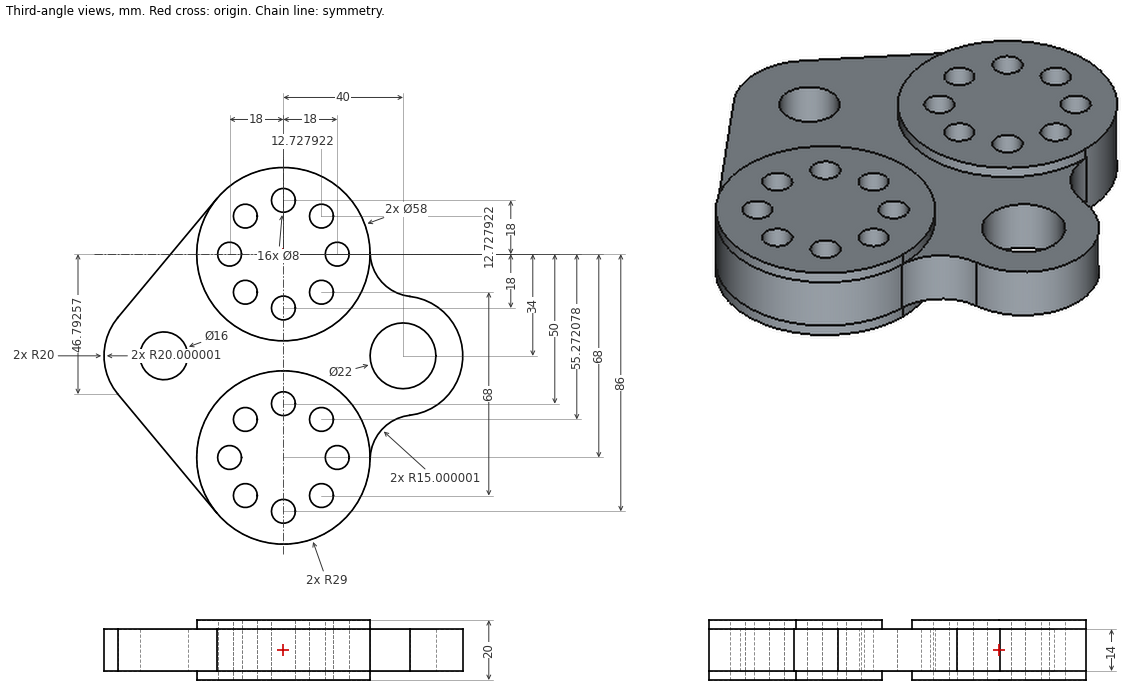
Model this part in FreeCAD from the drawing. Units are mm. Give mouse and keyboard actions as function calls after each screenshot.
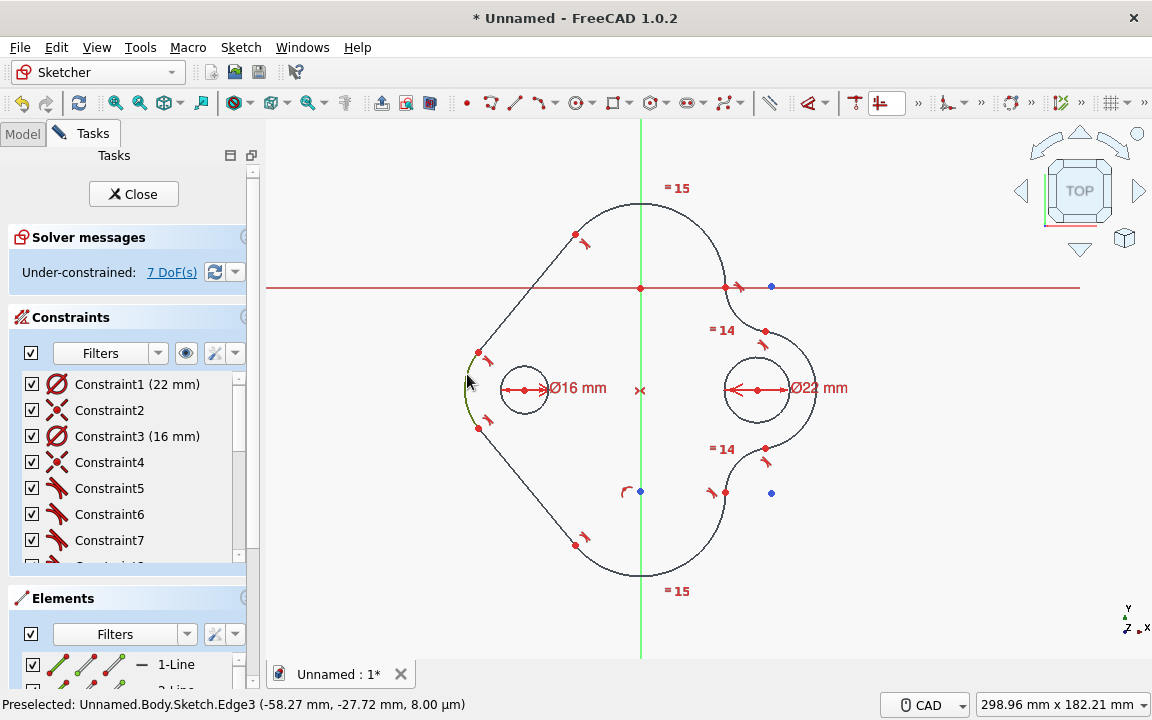
key(k)
key(r)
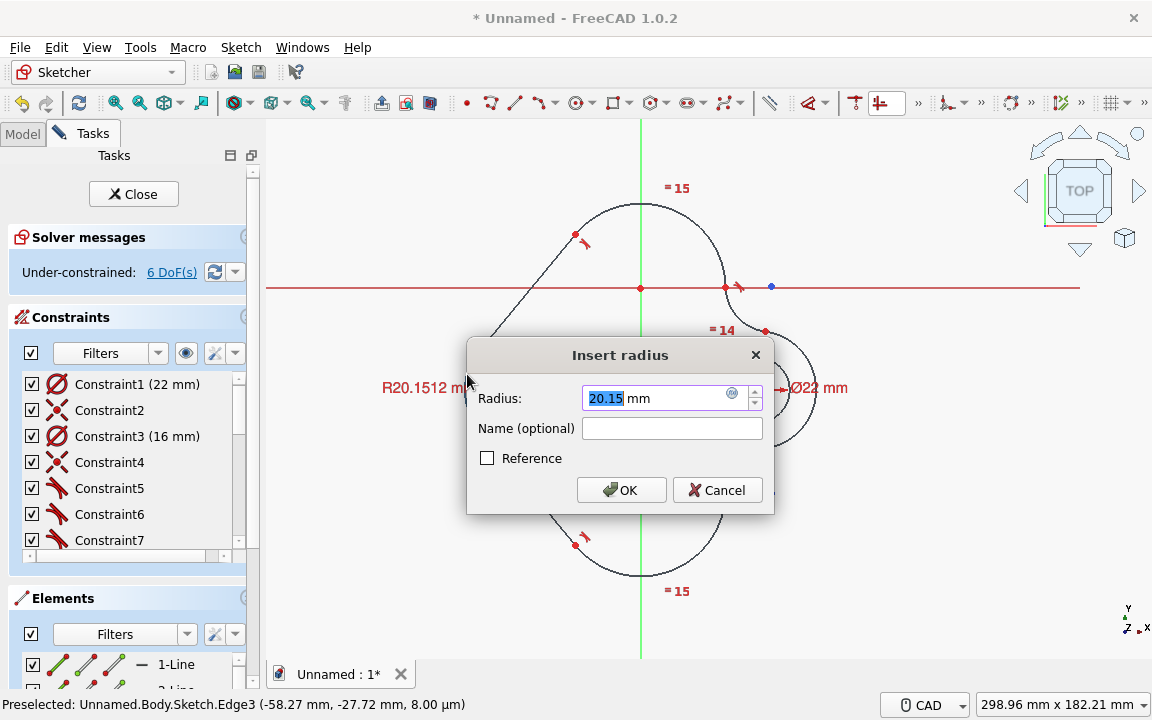
text(20.000001)
key(Return)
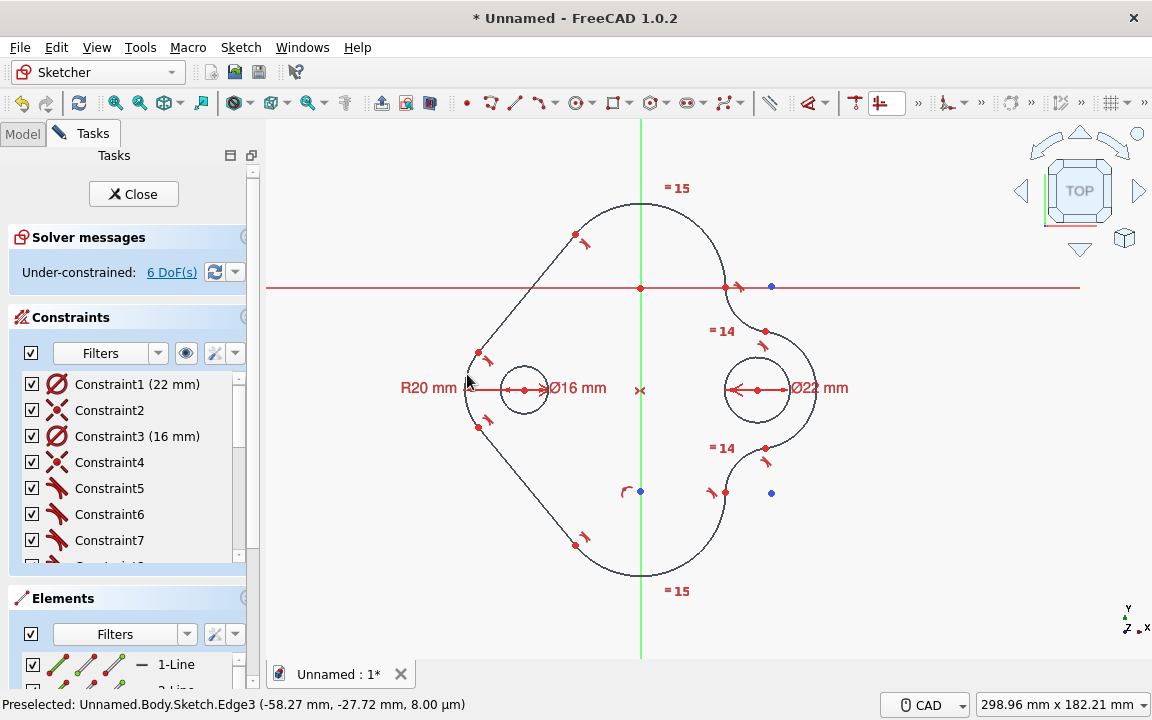
click(628, 575)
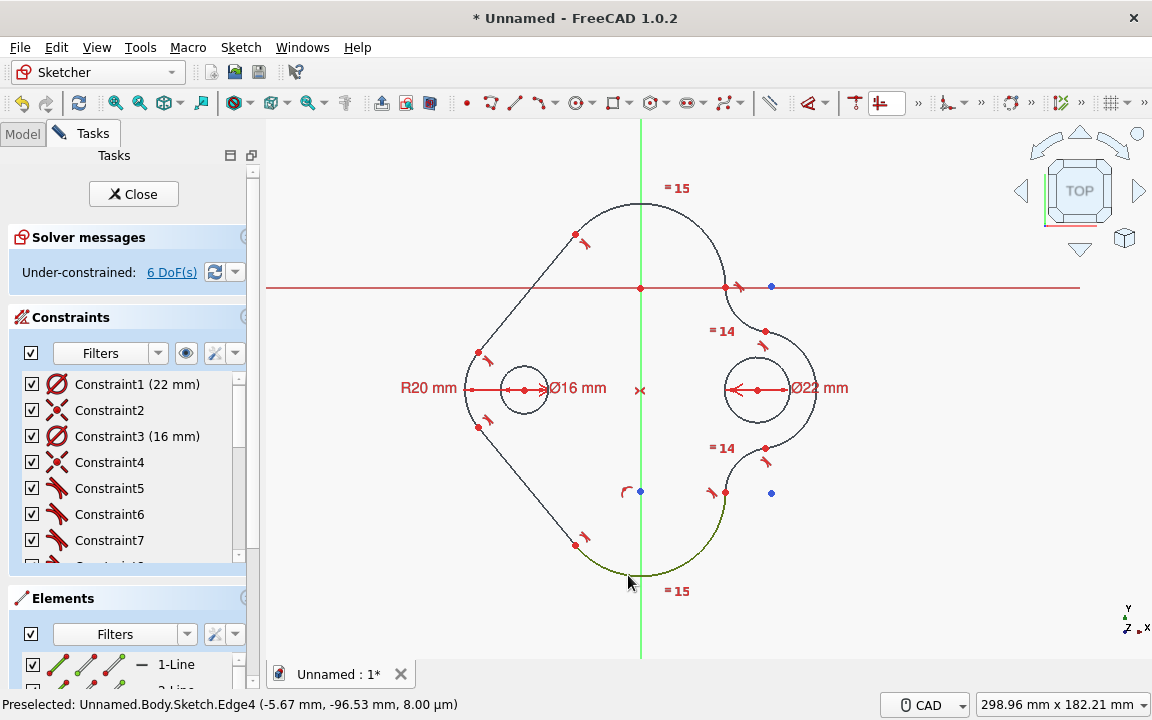
key(k)
key(r)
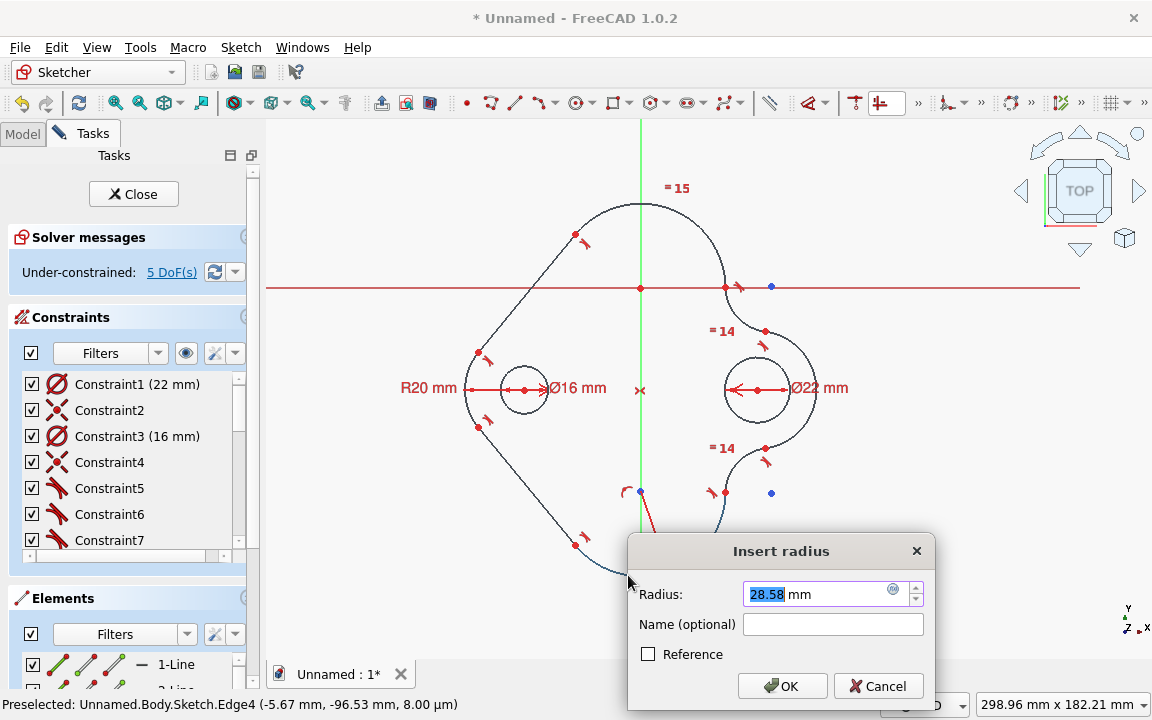
text(29)
key(Return)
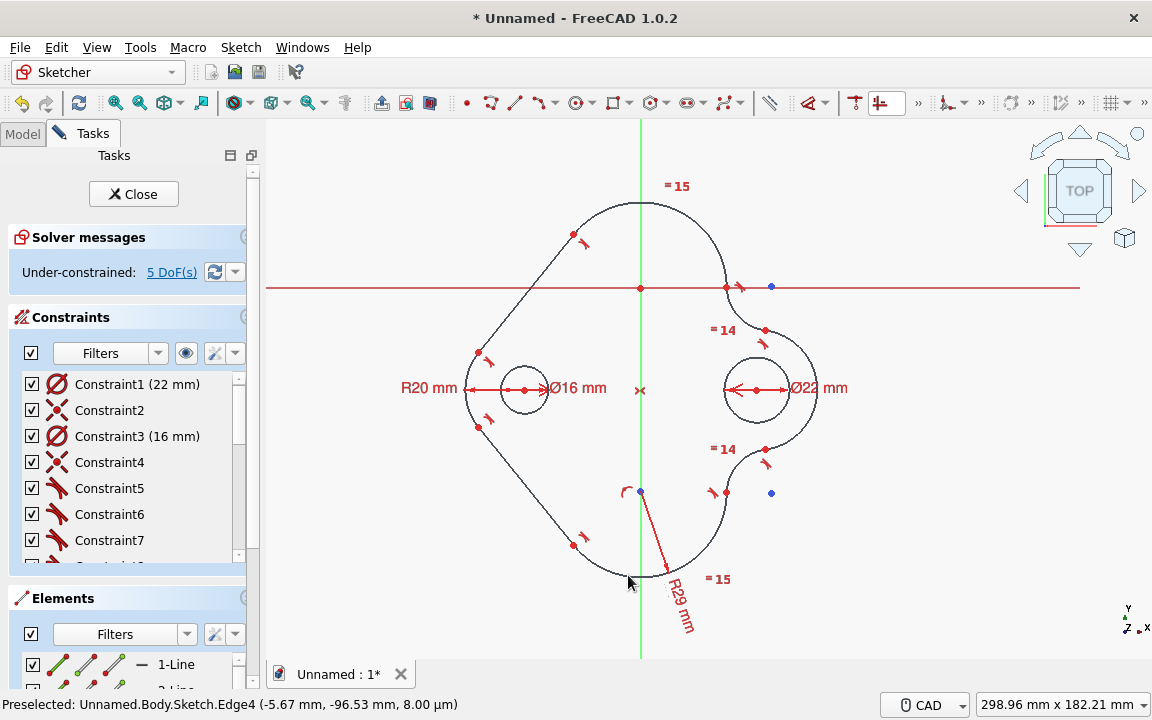
click(748, 456)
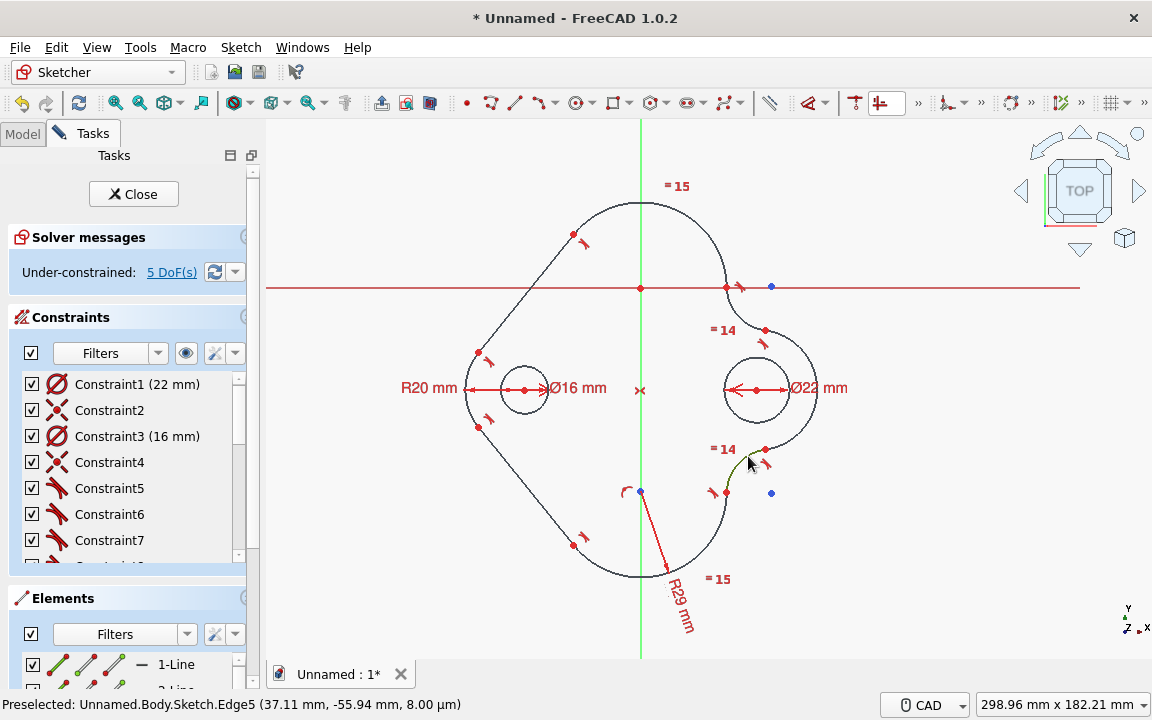
key(k)
key(r)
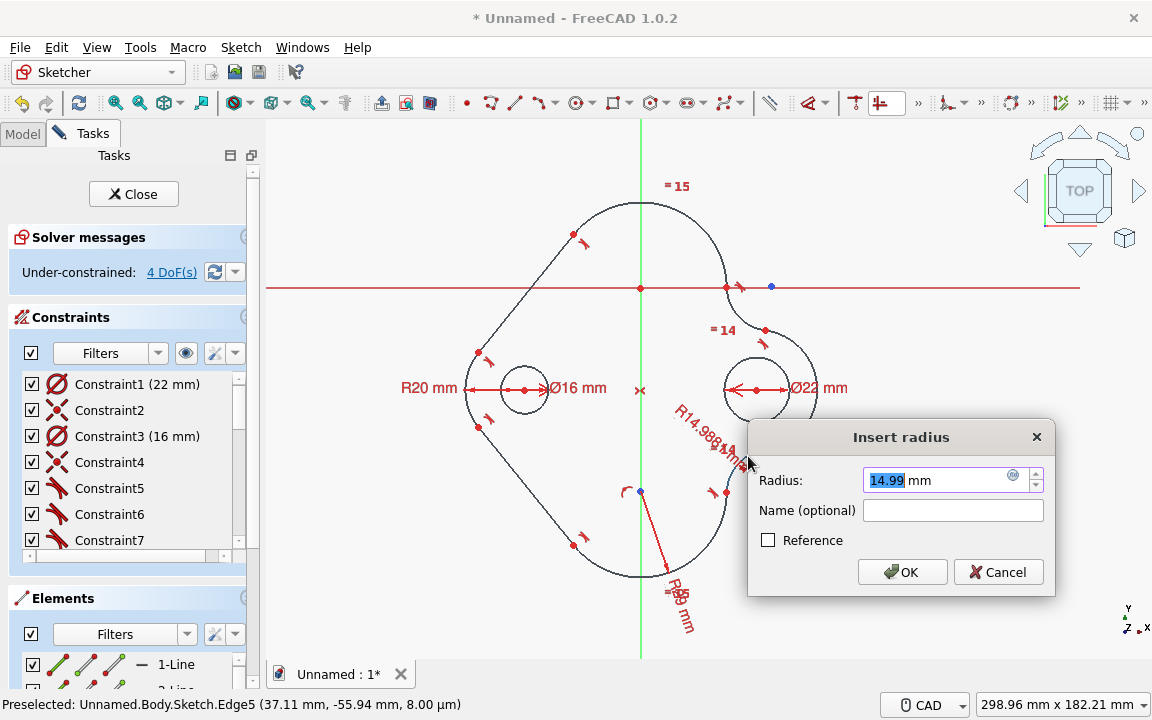
text(15.000001)
key(Return)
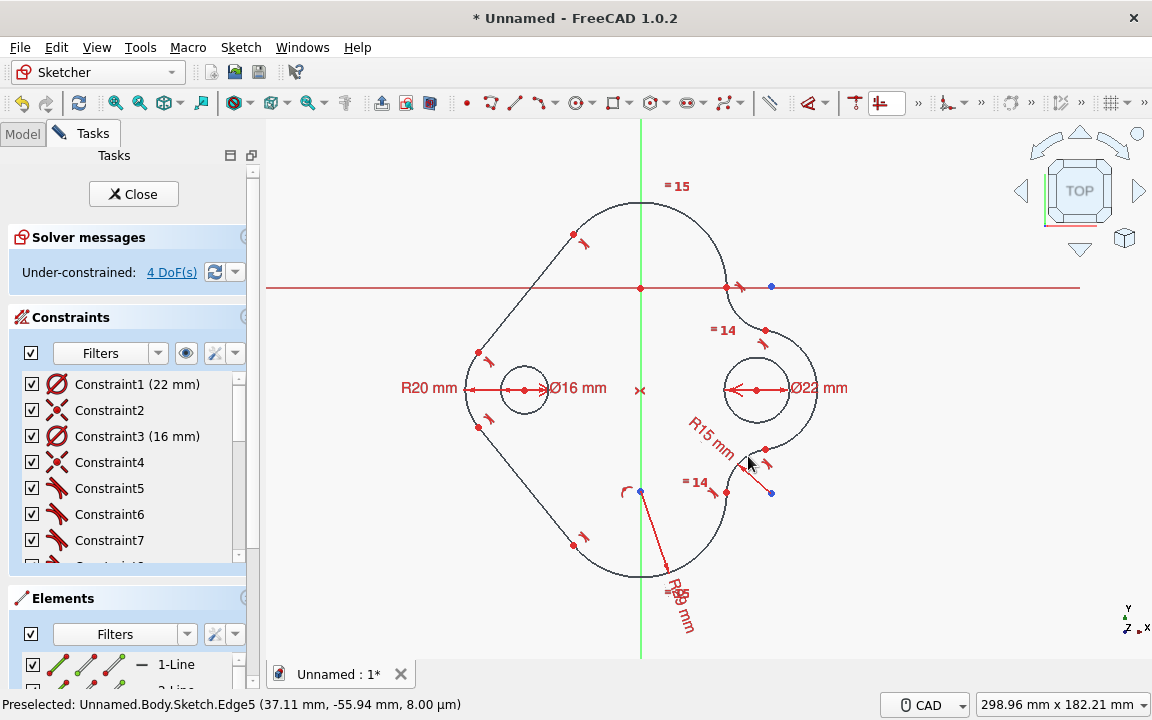
click(808, 423)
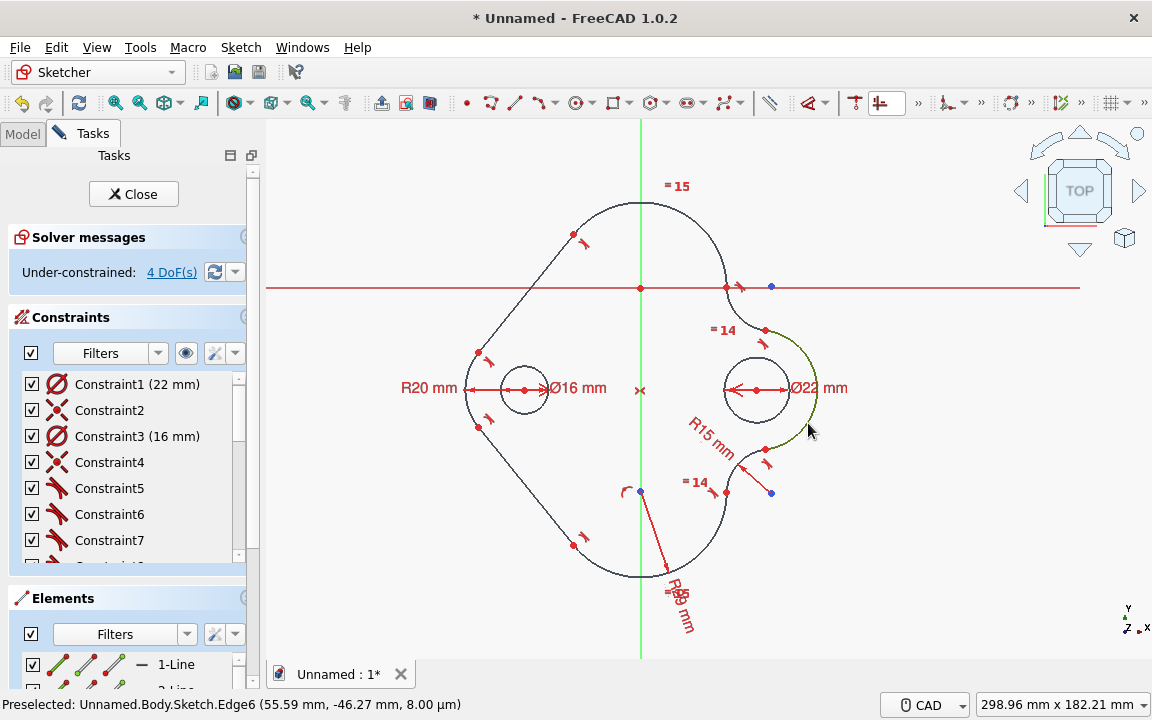
key(k)
key(r)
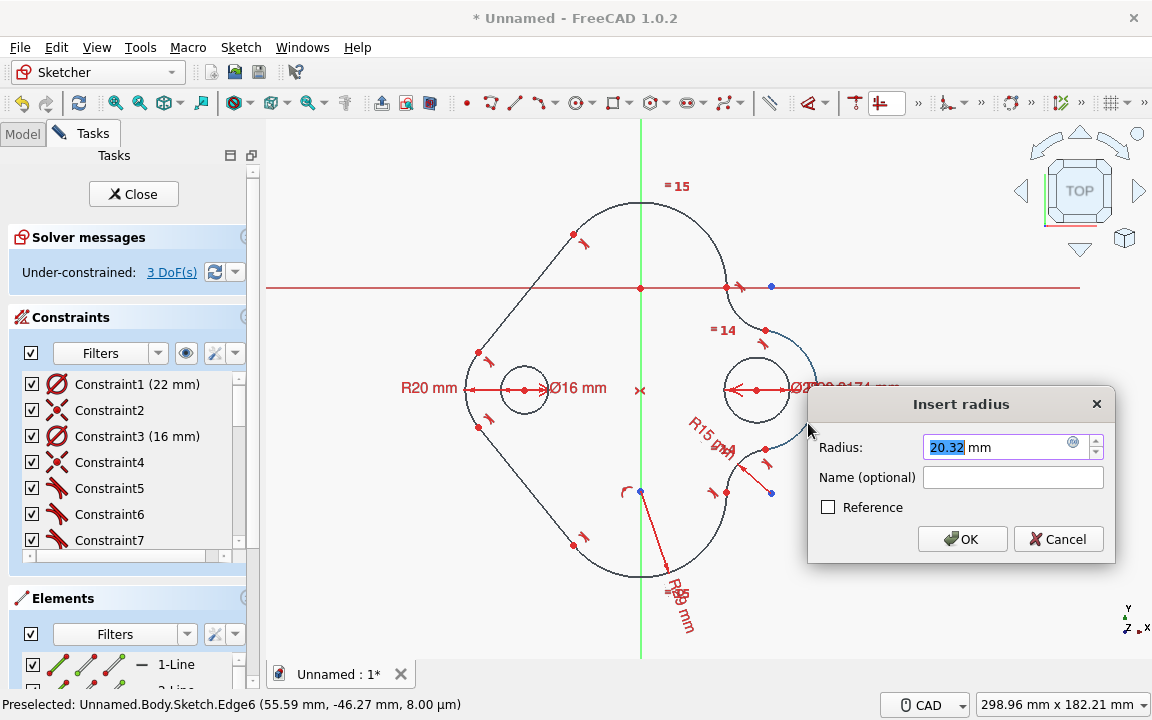
text(20)
key(Return)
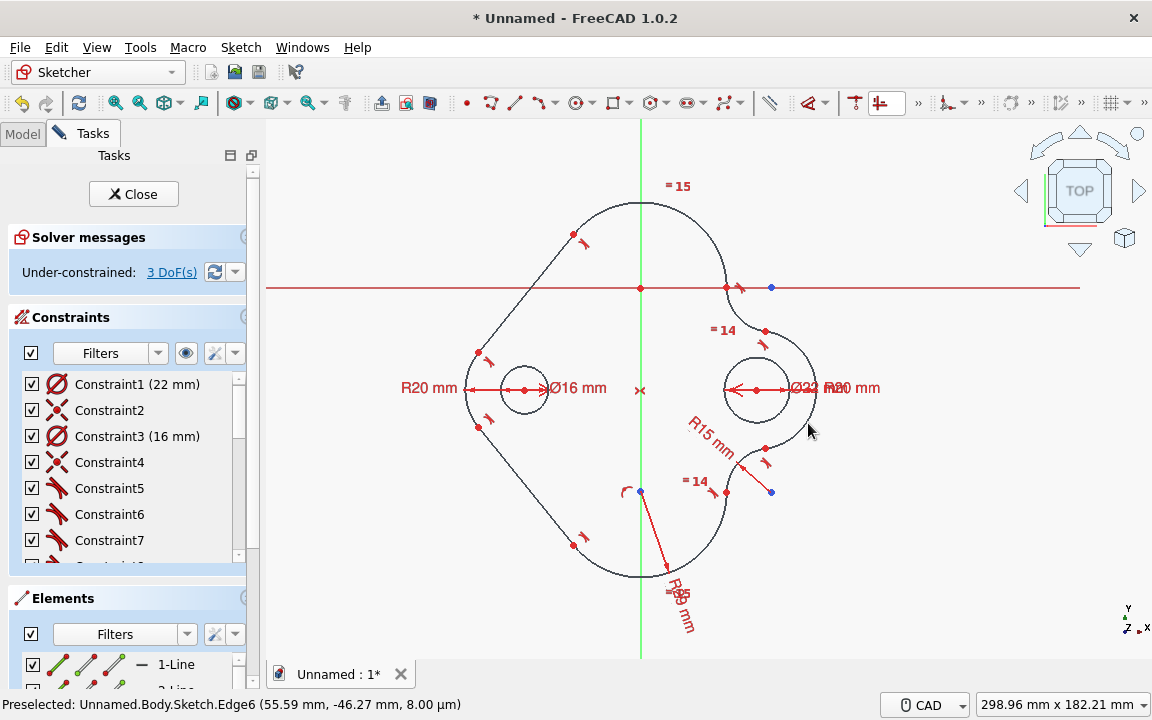
click(757, 390)